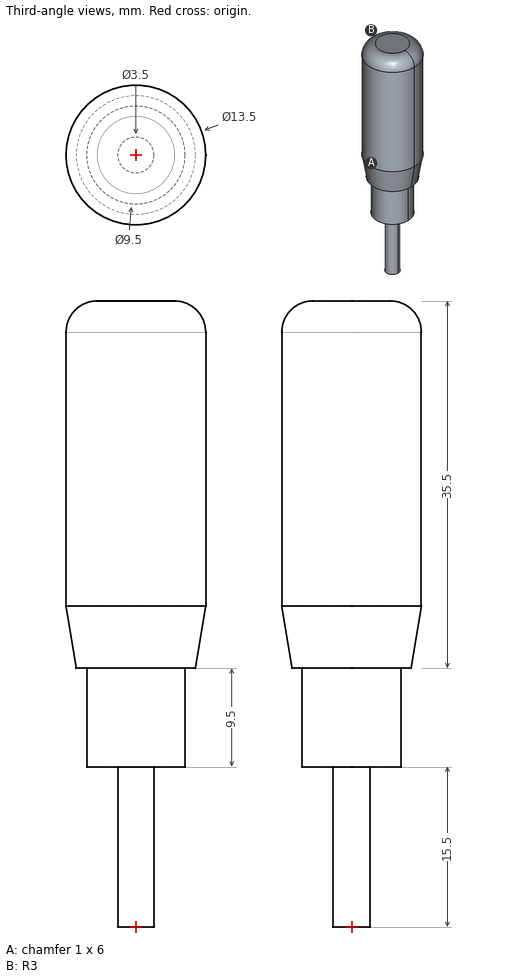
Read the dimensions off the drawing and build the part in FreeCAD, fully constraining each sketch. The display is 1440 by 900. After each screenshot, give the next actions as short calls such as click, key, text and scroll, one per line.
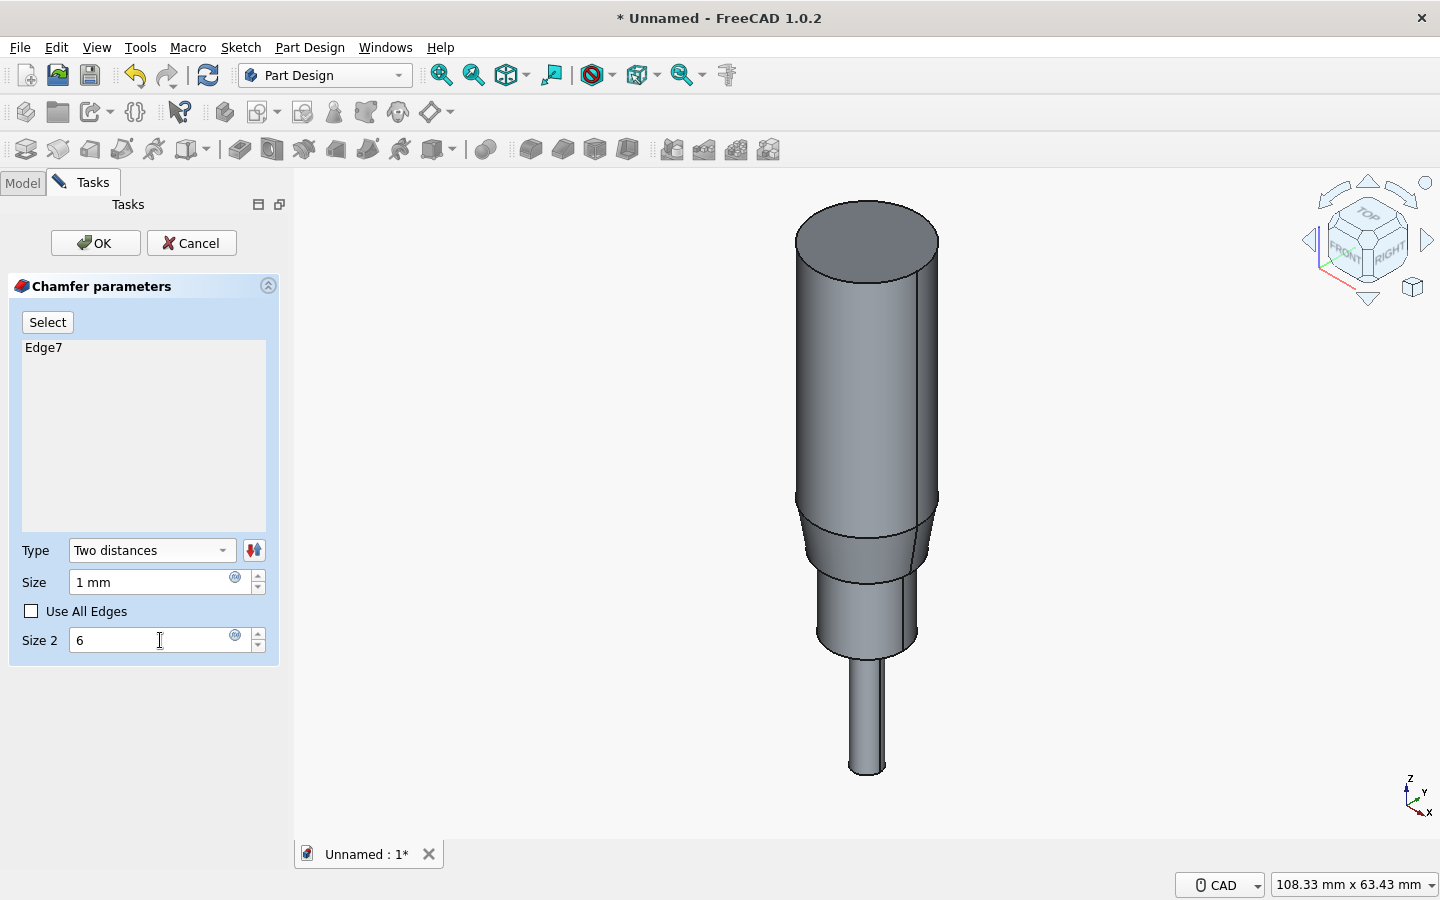
click(96, 243)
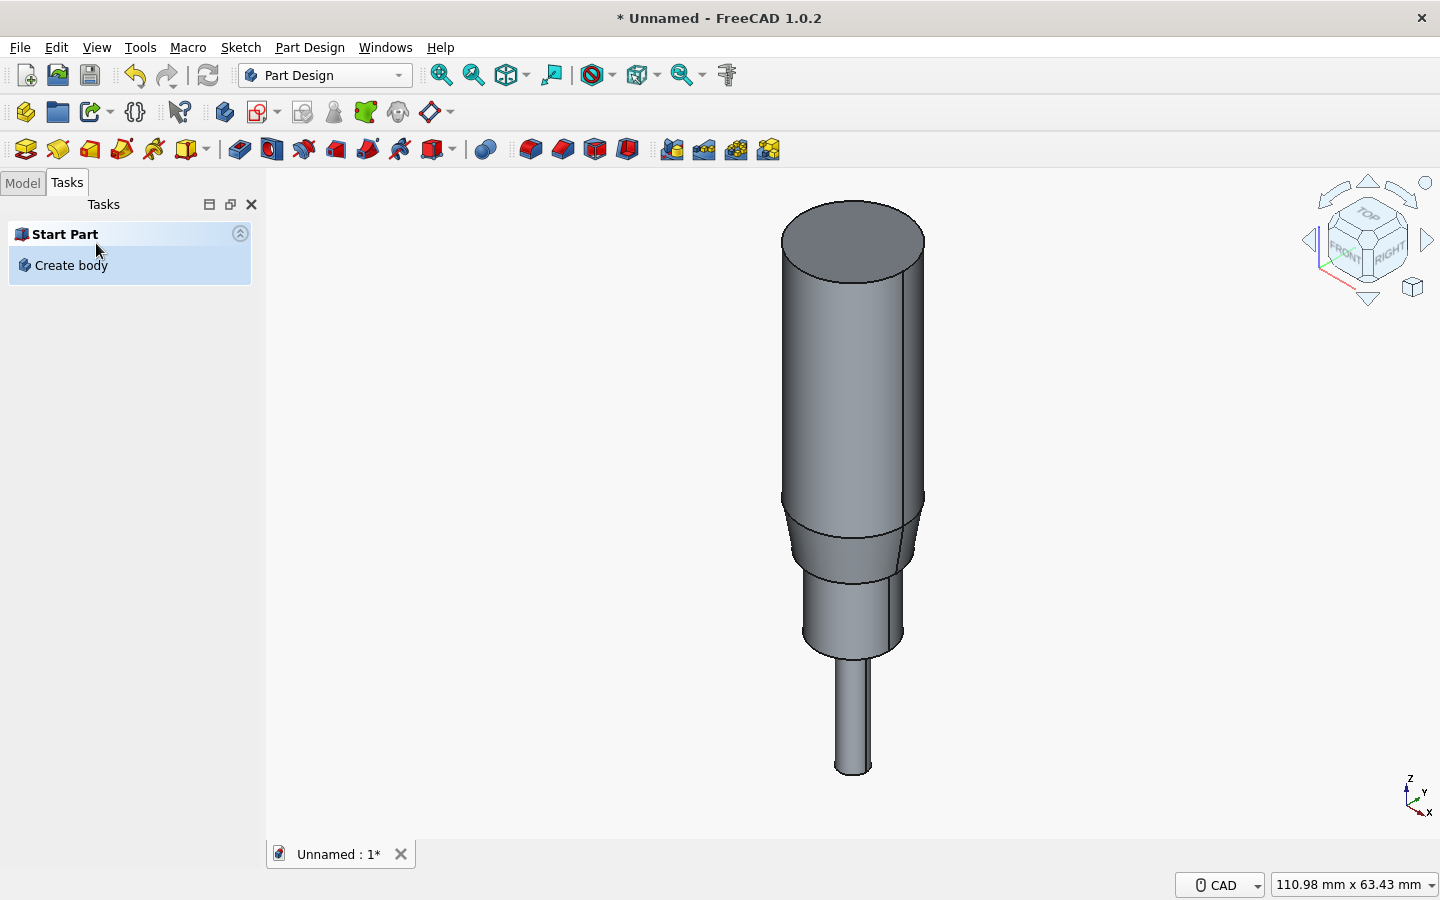
click(885, 204)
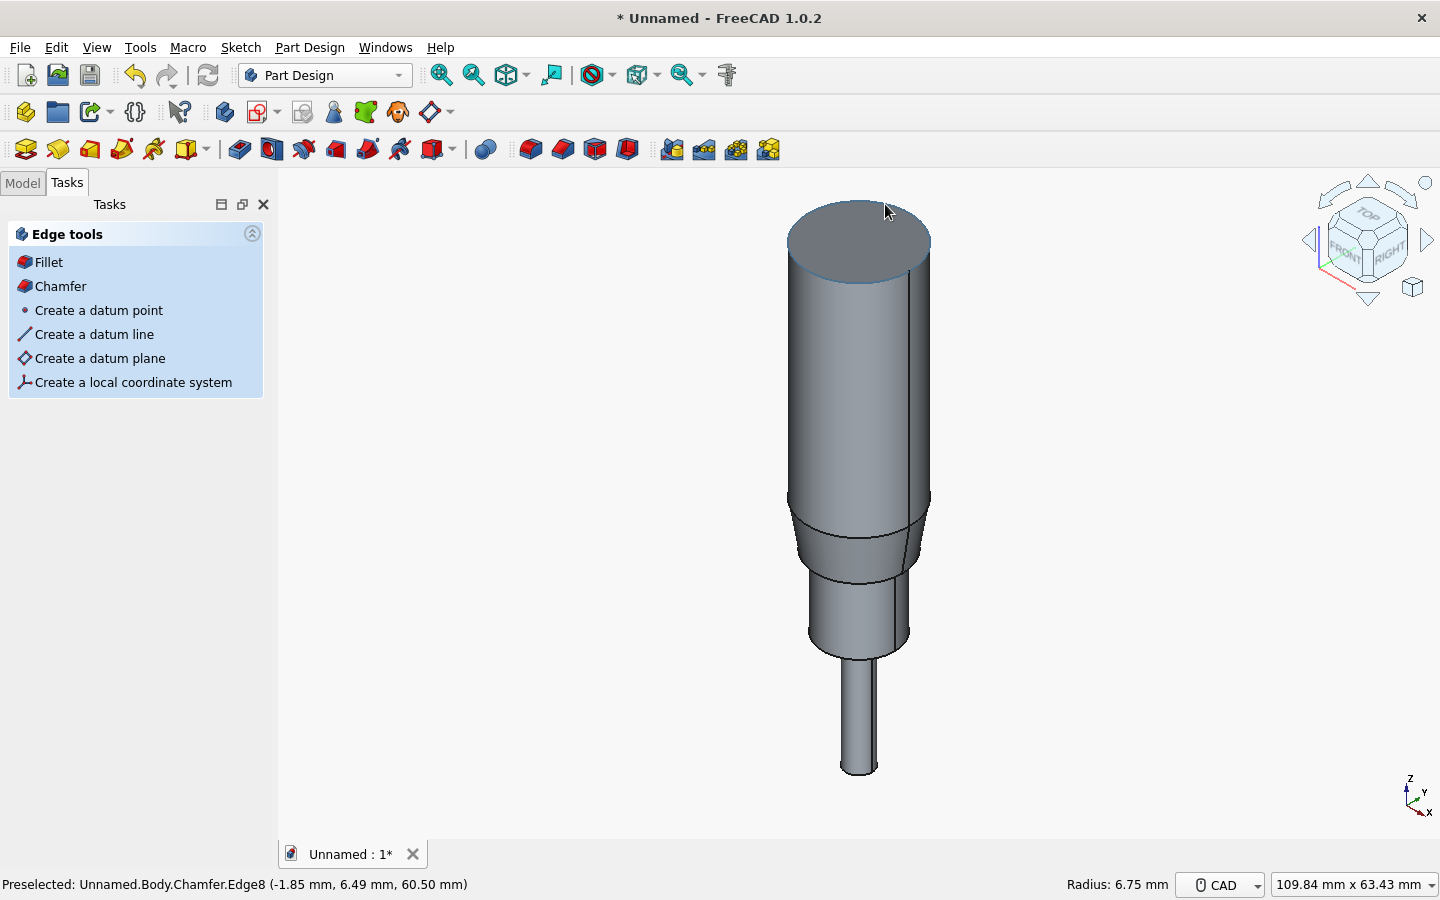
click(532, 150)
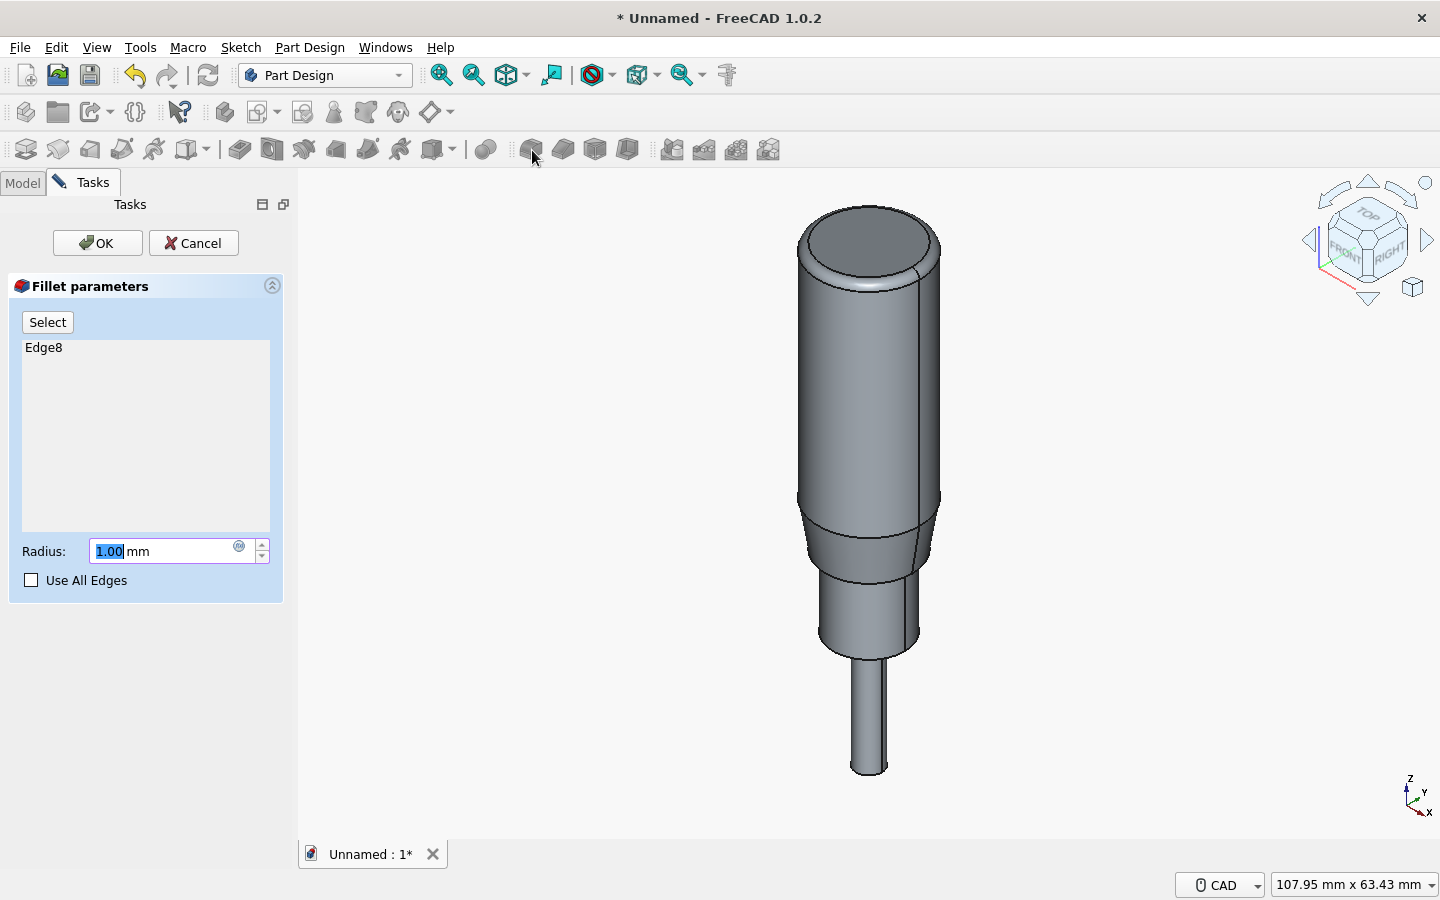
text(3)
key(Tab)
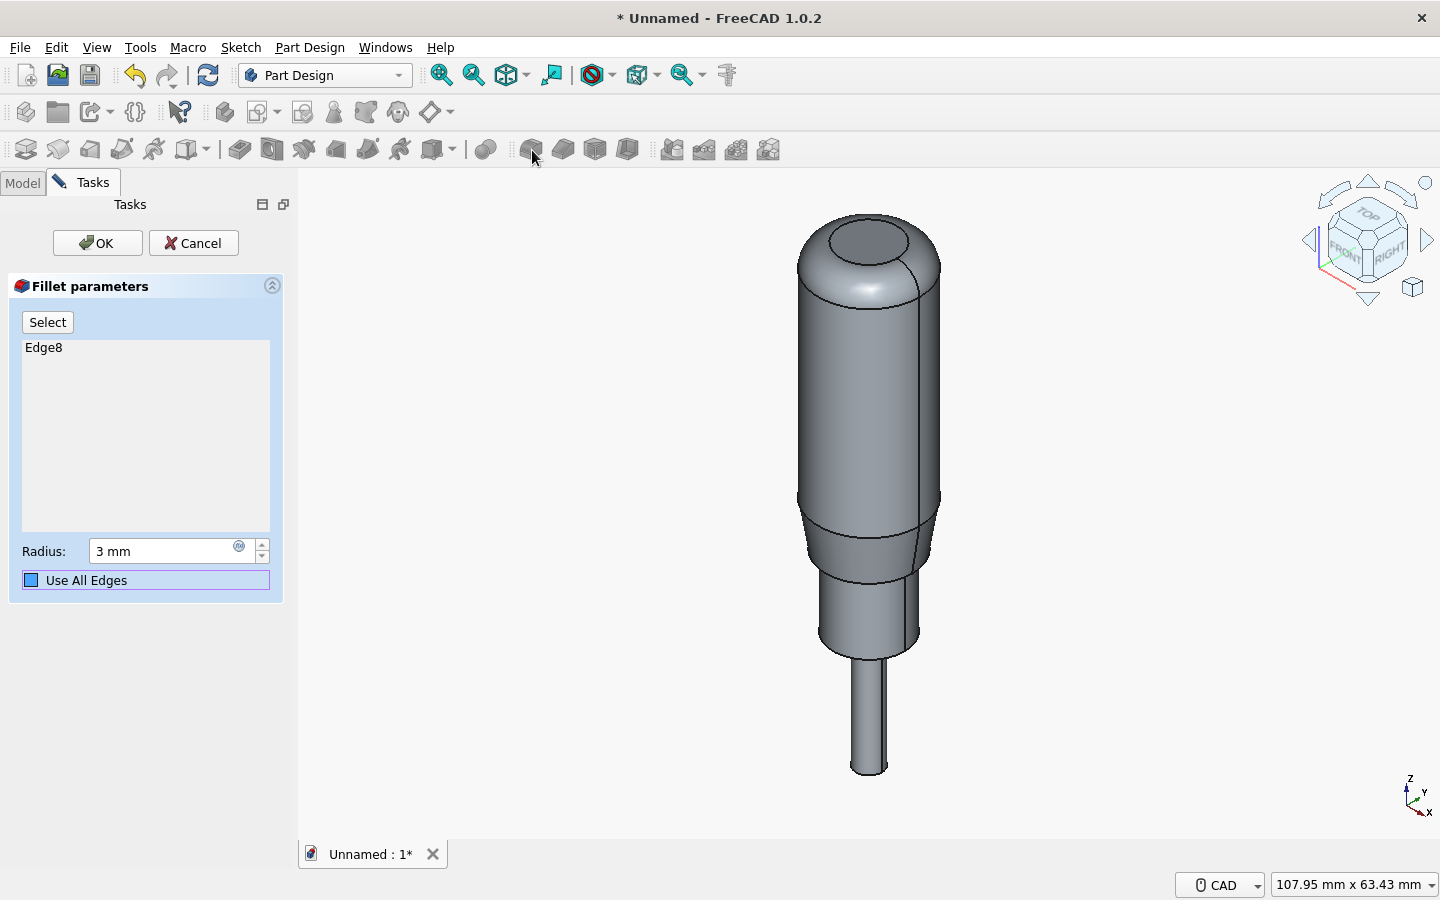
click(98, 243)